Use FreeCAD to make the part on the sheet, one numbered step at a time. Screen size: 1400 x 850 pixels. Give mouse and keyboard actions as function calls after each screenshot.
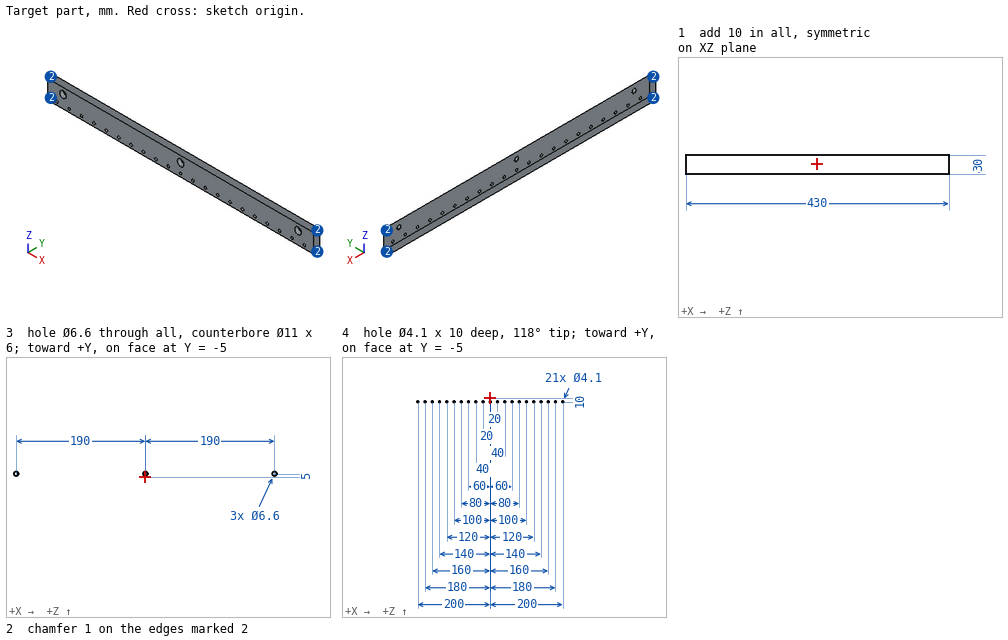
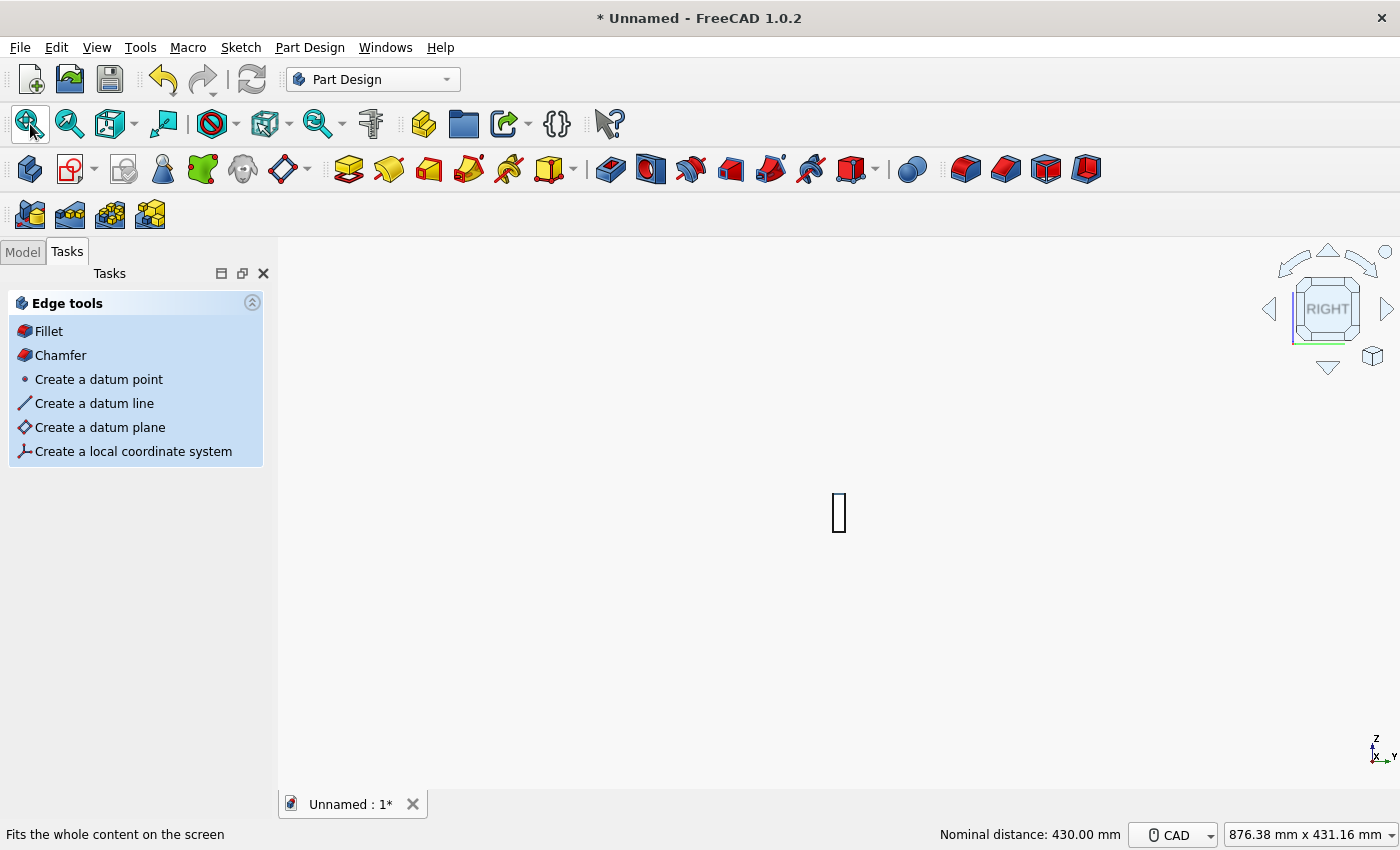
click(30, 124)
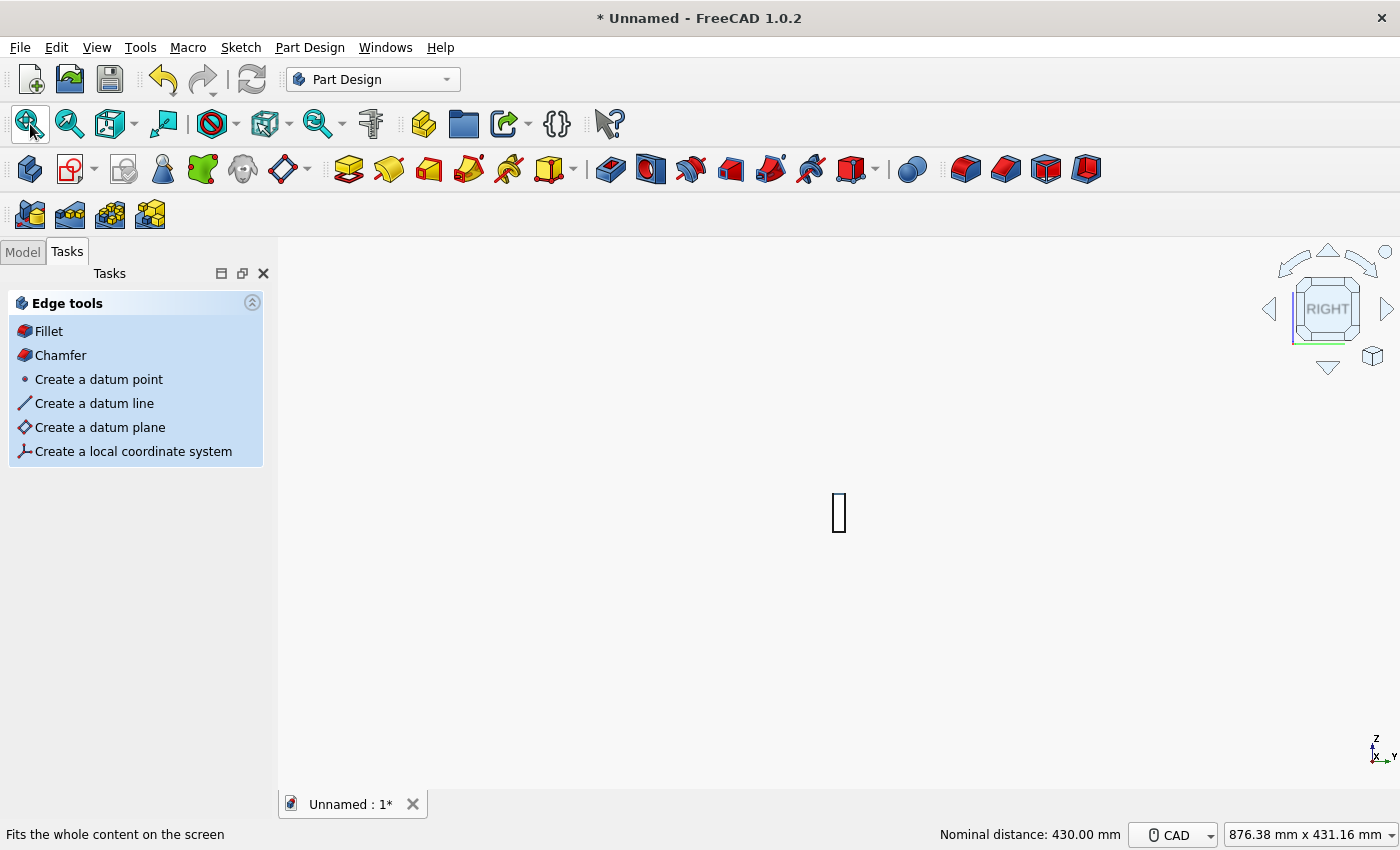
click(839, 531, ctrl)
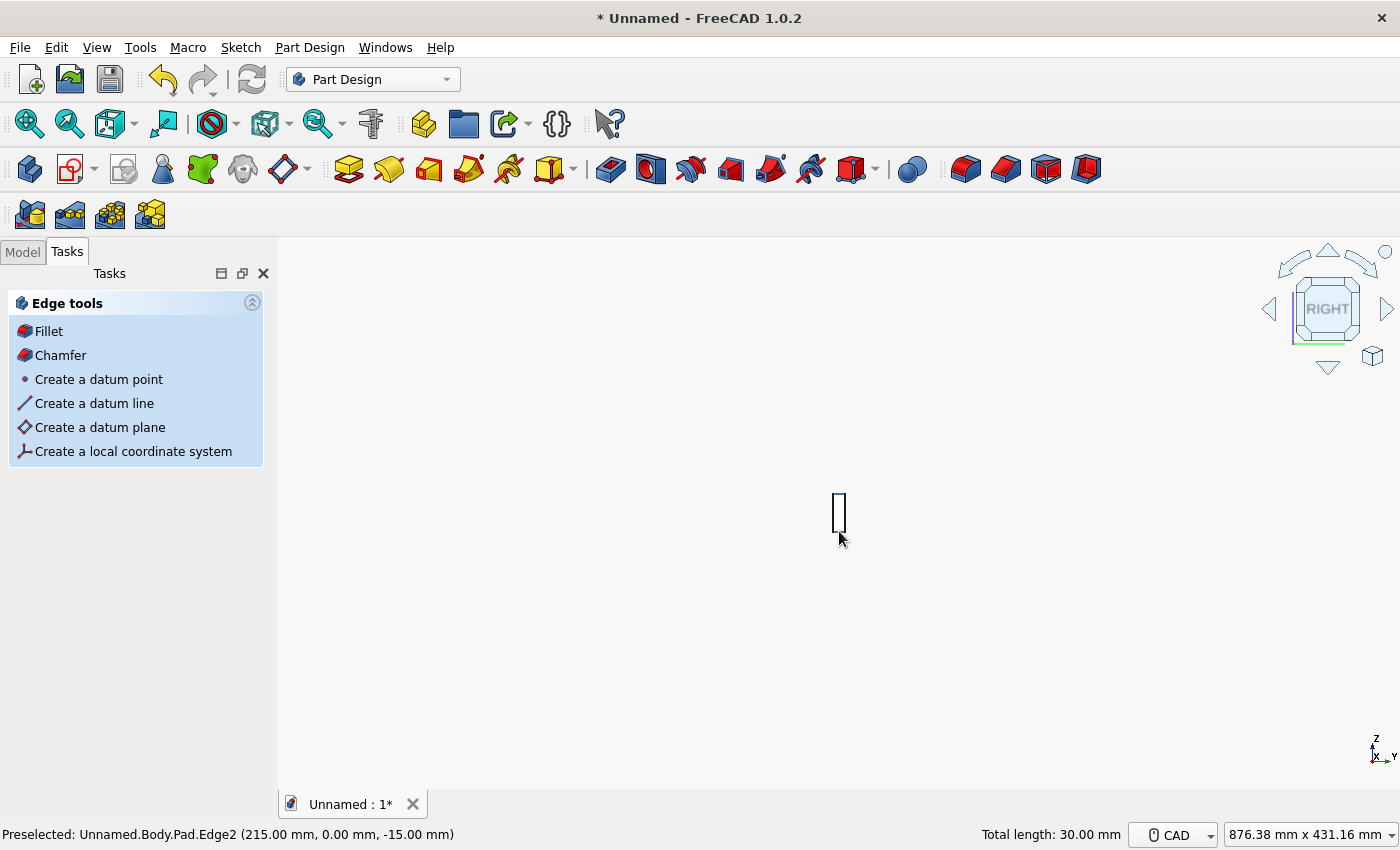
scroll(839, 531, up, 6)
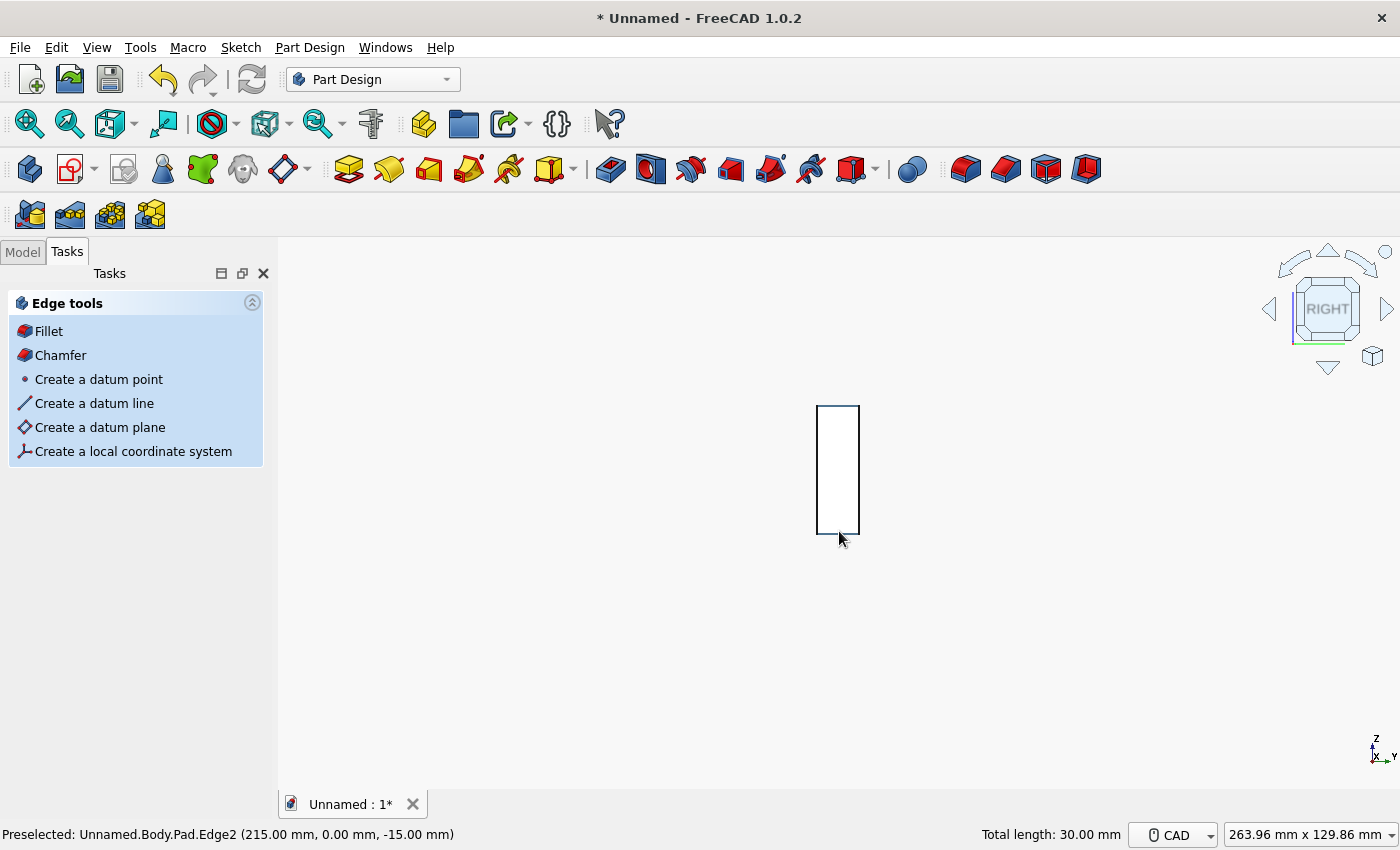
click(30, 124)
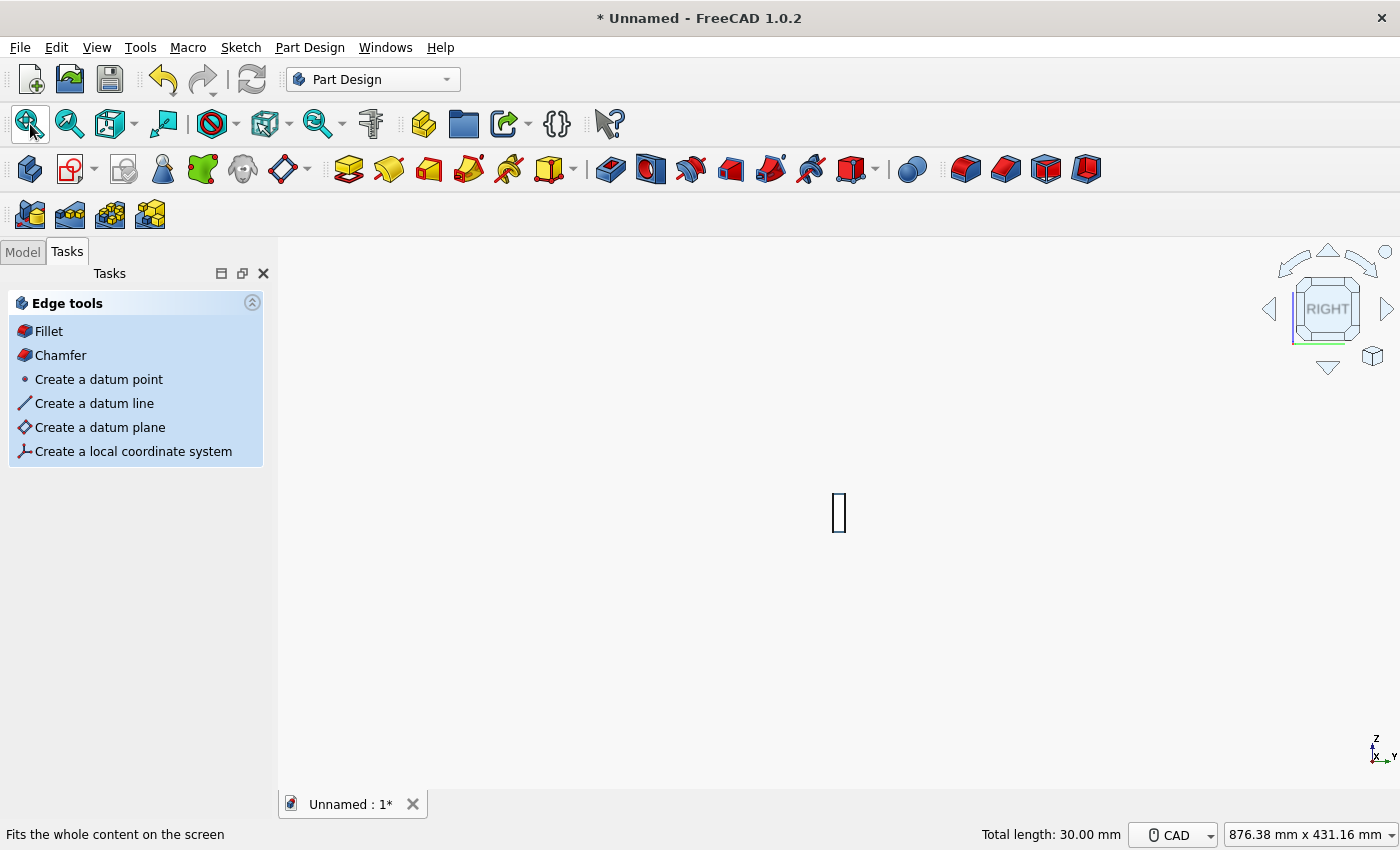
key(5)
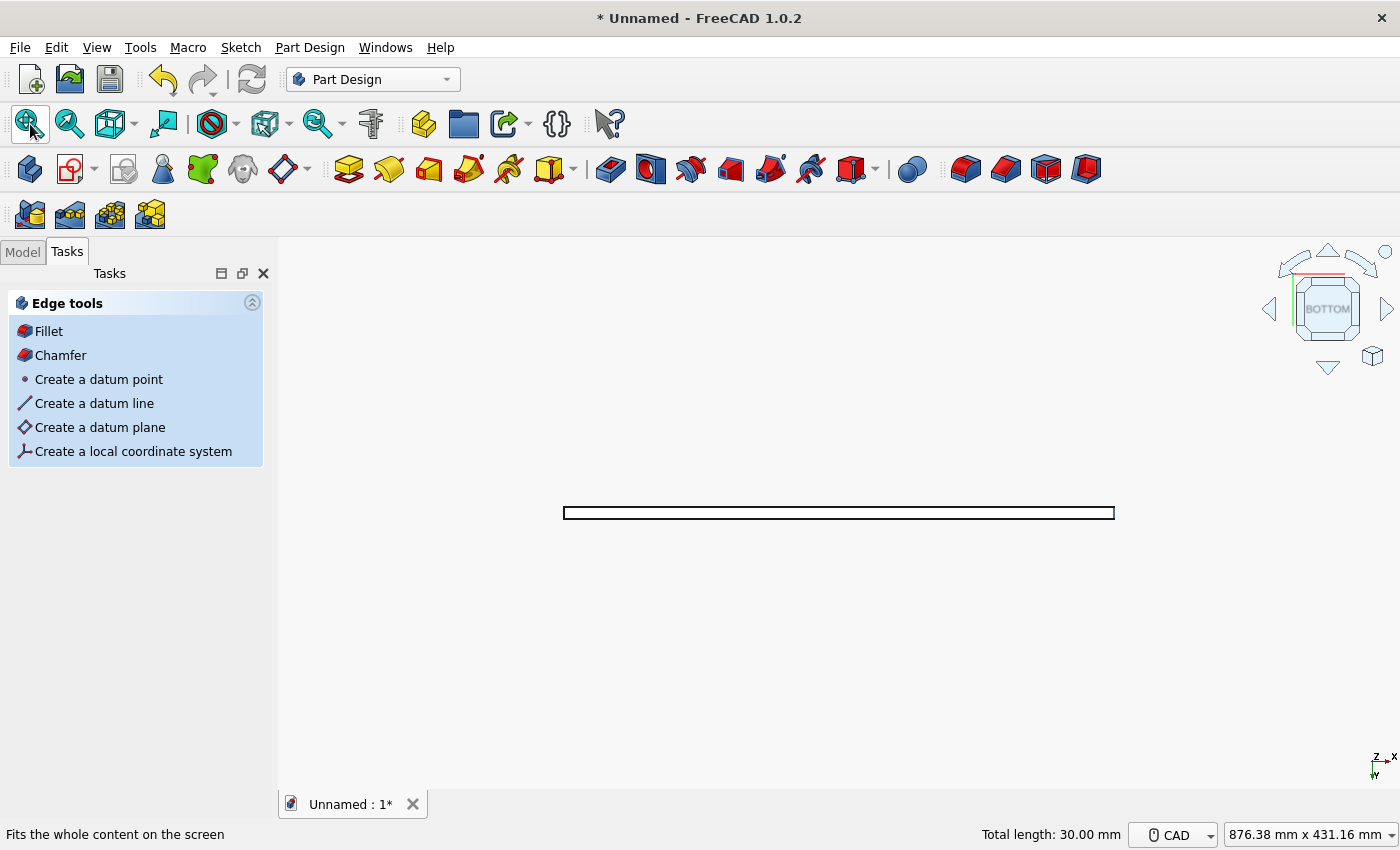
click(564, 512, ctrl)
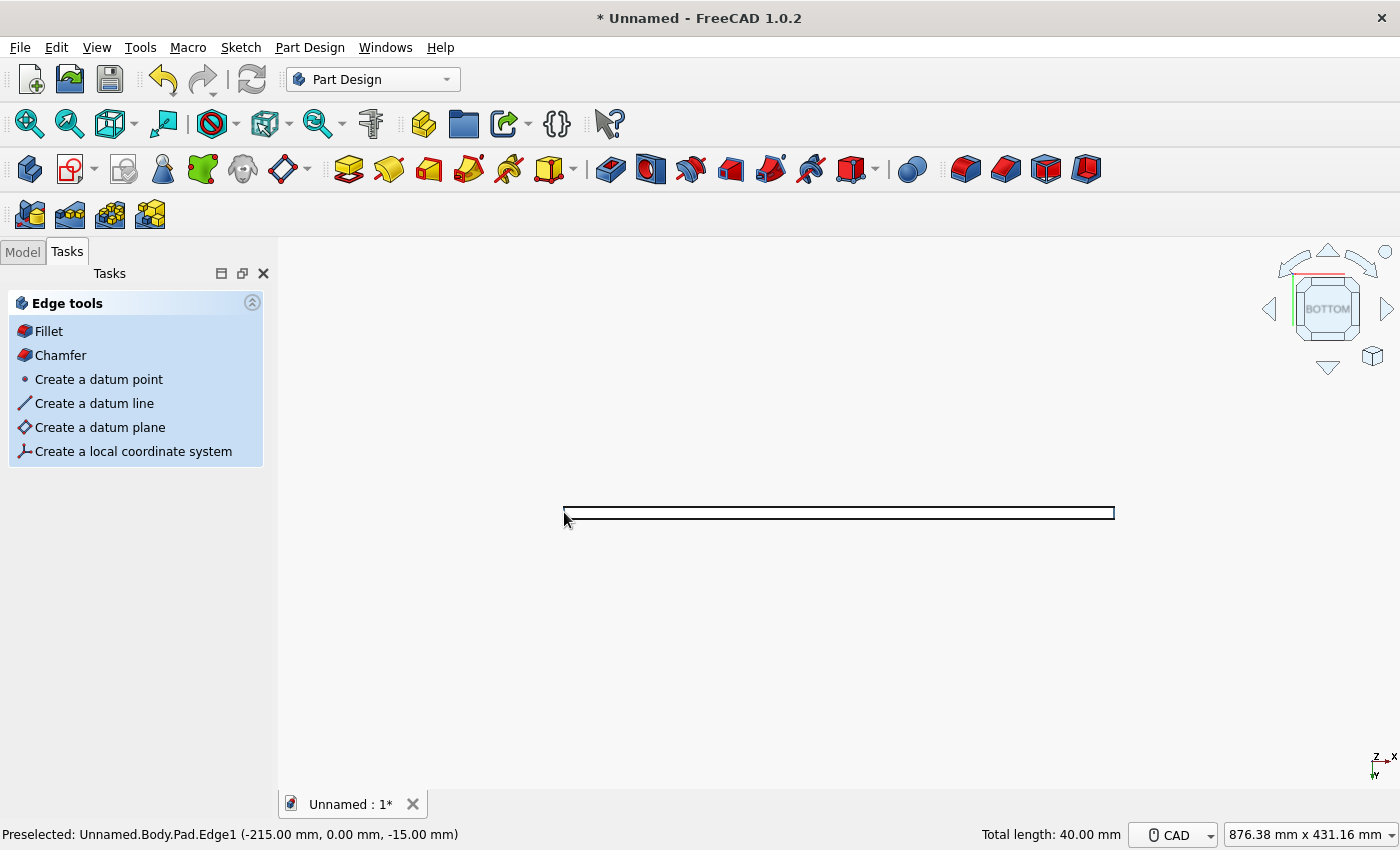
click(1006, 170)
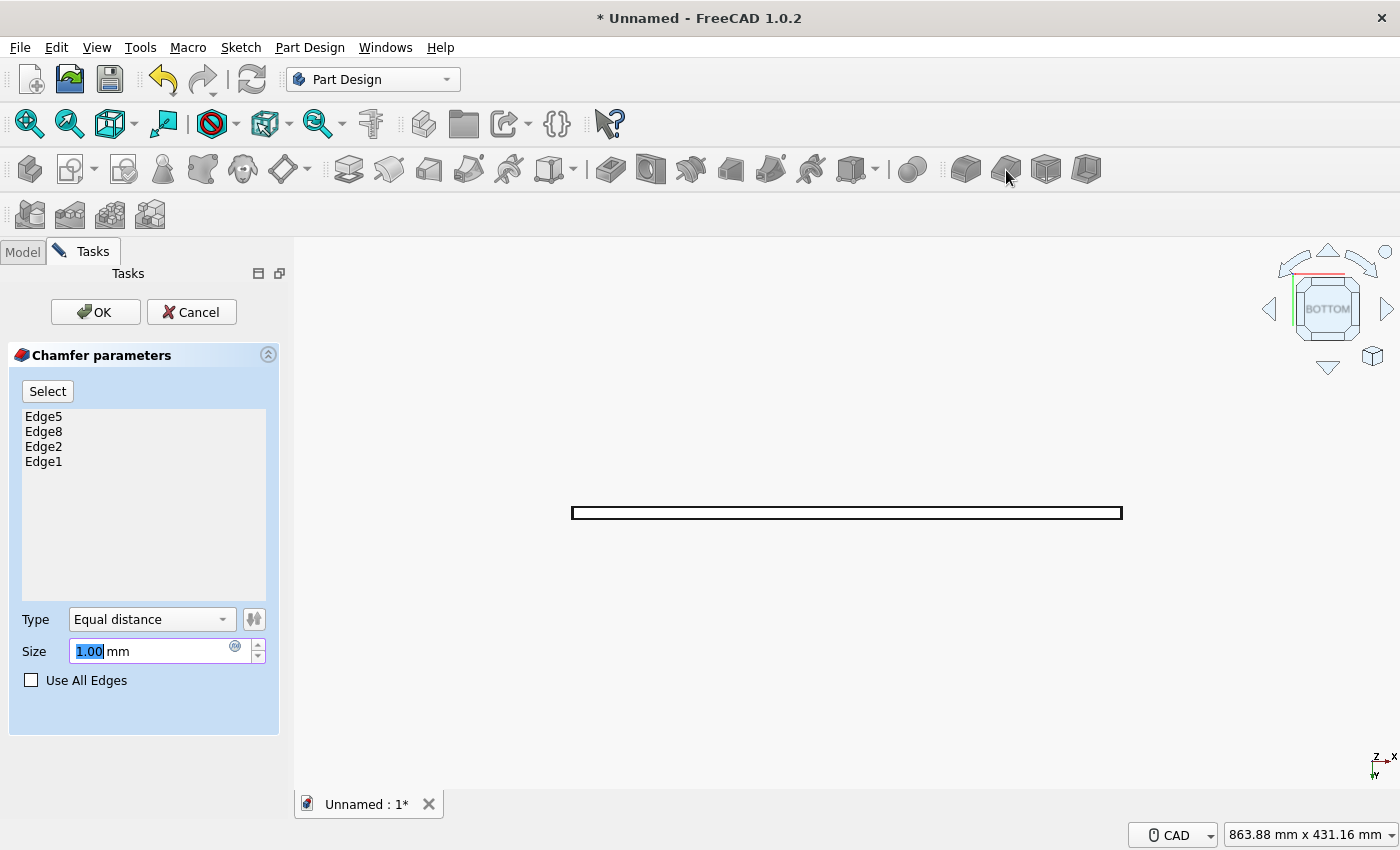
text(1)
key(Tab)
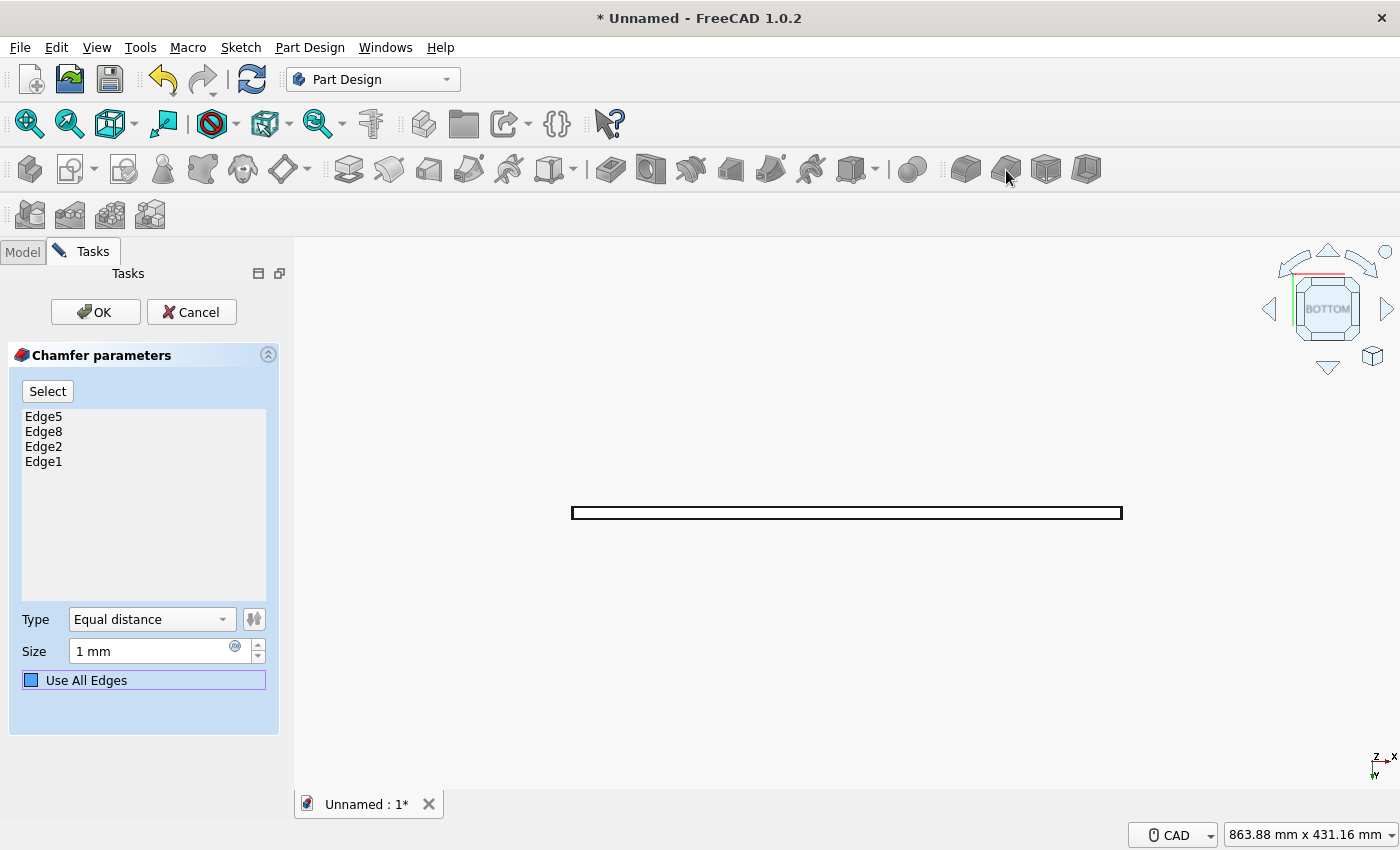
click(96, 312)